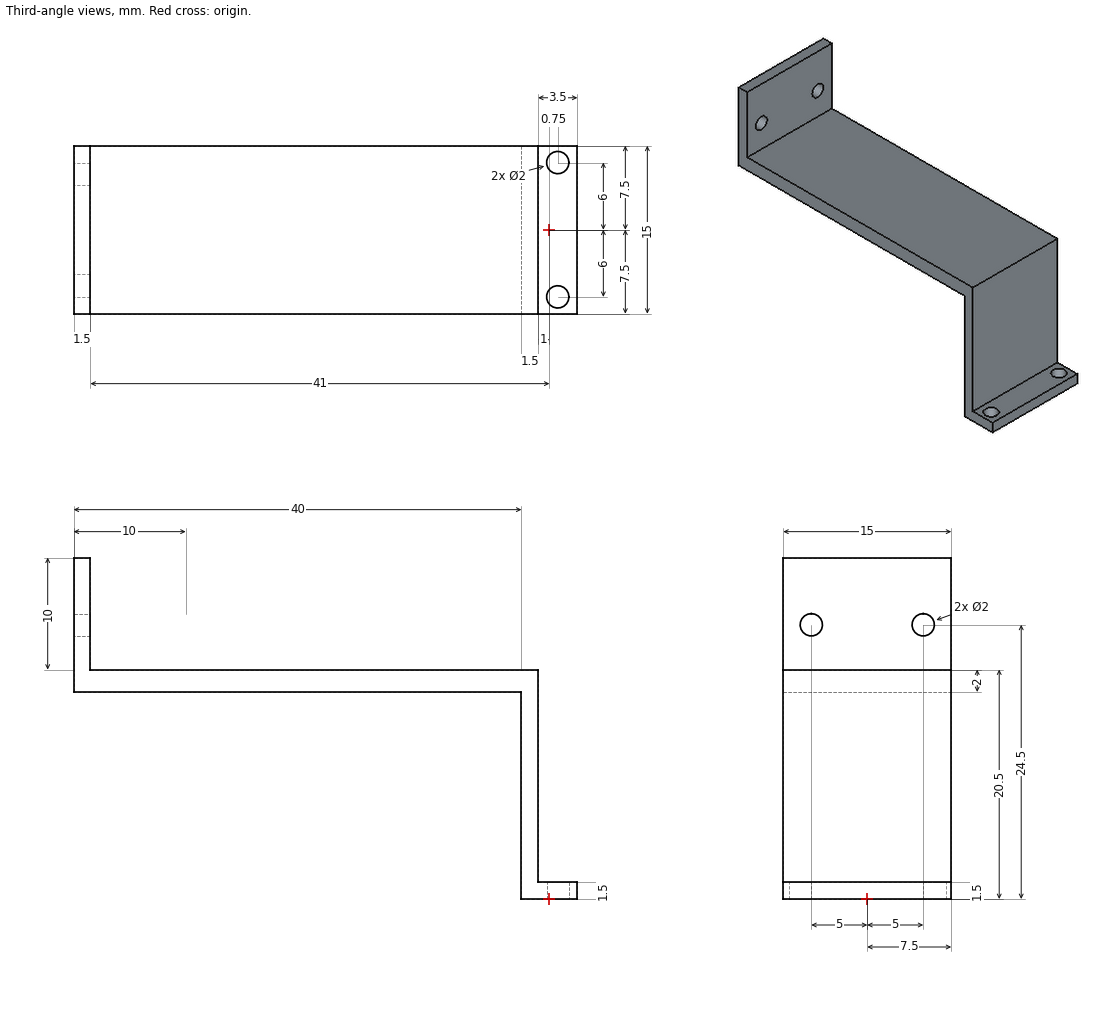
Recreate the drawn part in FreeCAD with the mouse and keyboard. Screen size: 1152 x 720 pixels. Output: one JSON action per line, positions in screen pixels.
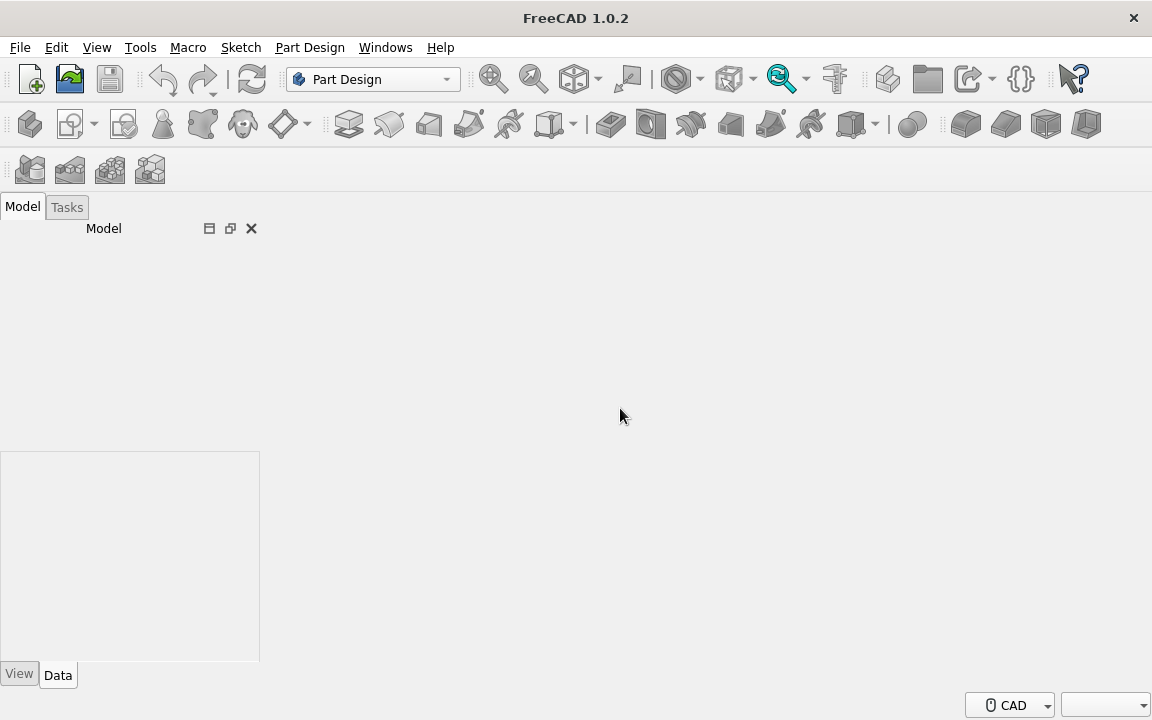
{"action": "left_click", "coordinate": [30, 80]}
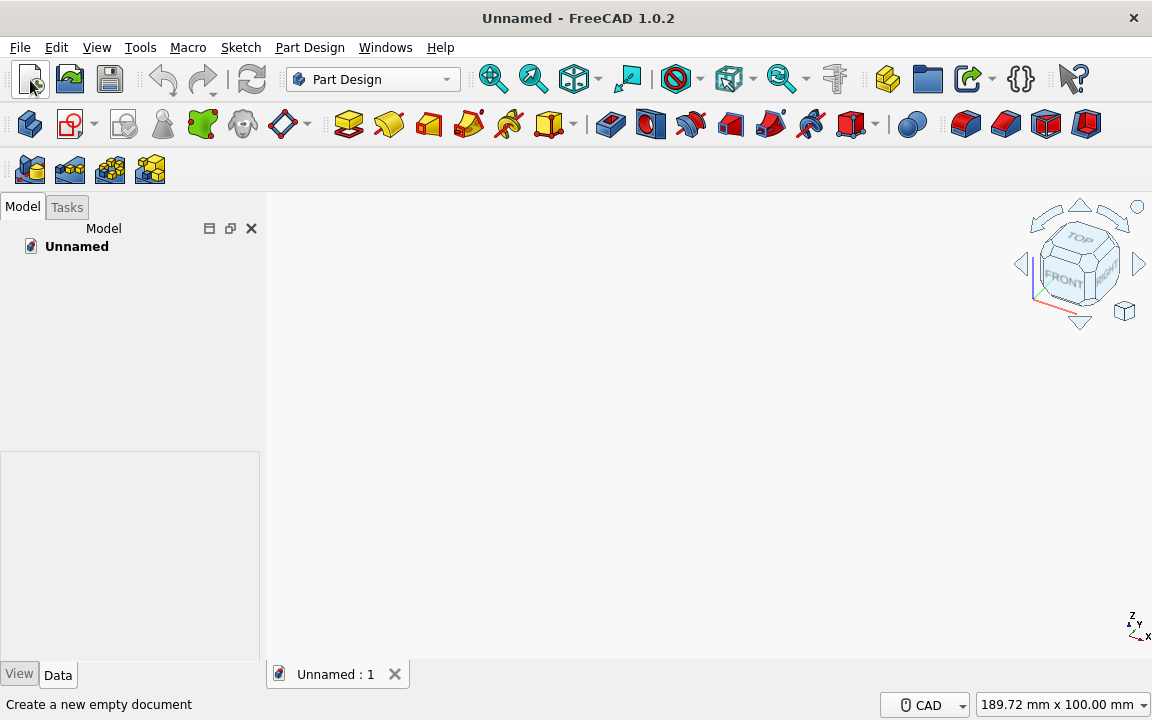
{"action": "left_click", "coordinate": [70, 124]}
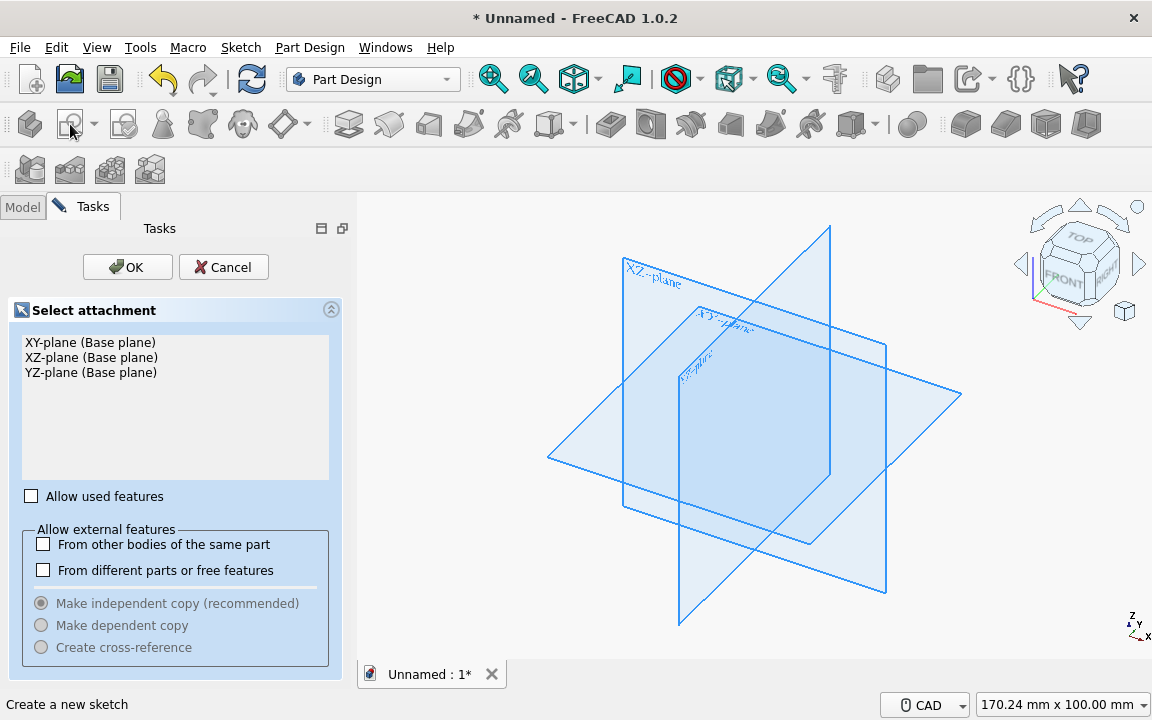
{"action": "left_click", "coordinate": [82, 342]}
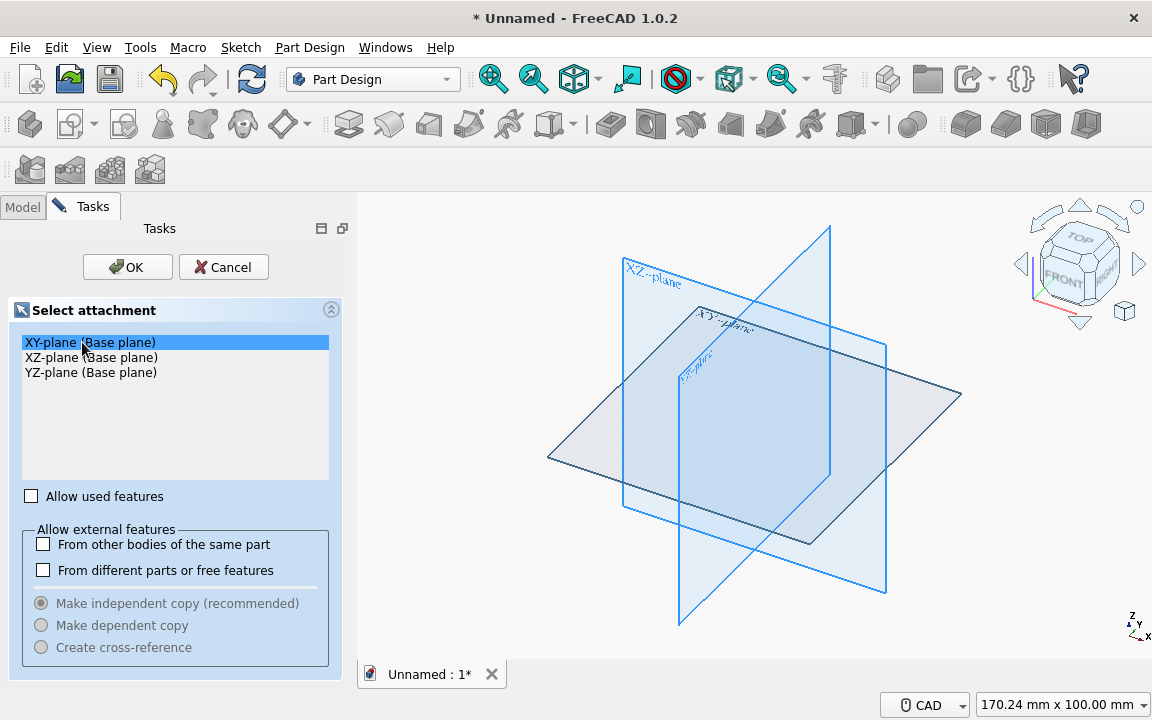
{"action": "left_click", "coordinate": [128, 267]}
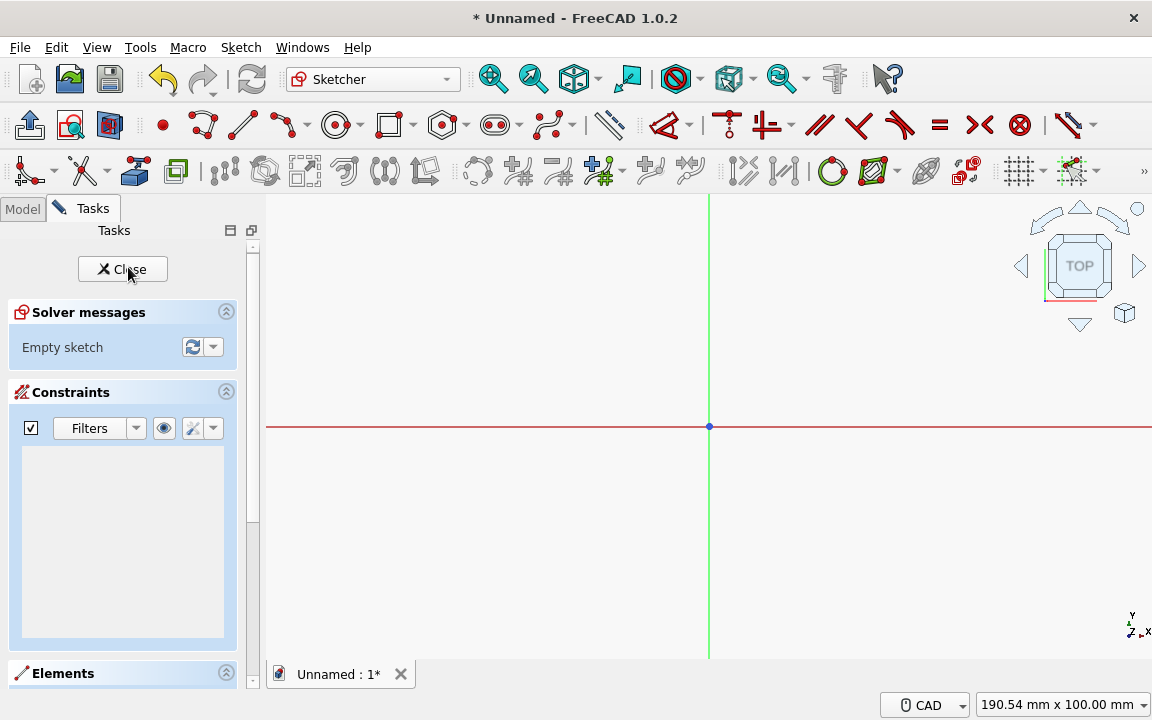
{"action": "scroll", "coordinate": [724, 426], "scroll_direction": "up", "scroll_amount": 7}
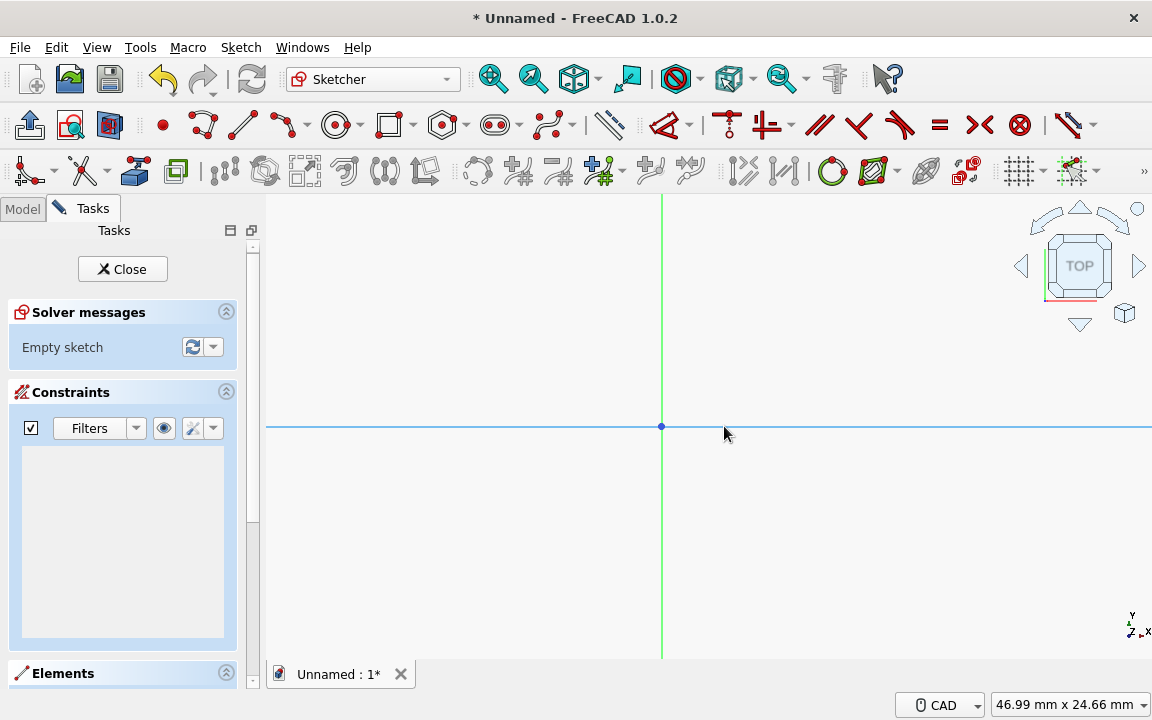
{"action": "key", "text": "g r"}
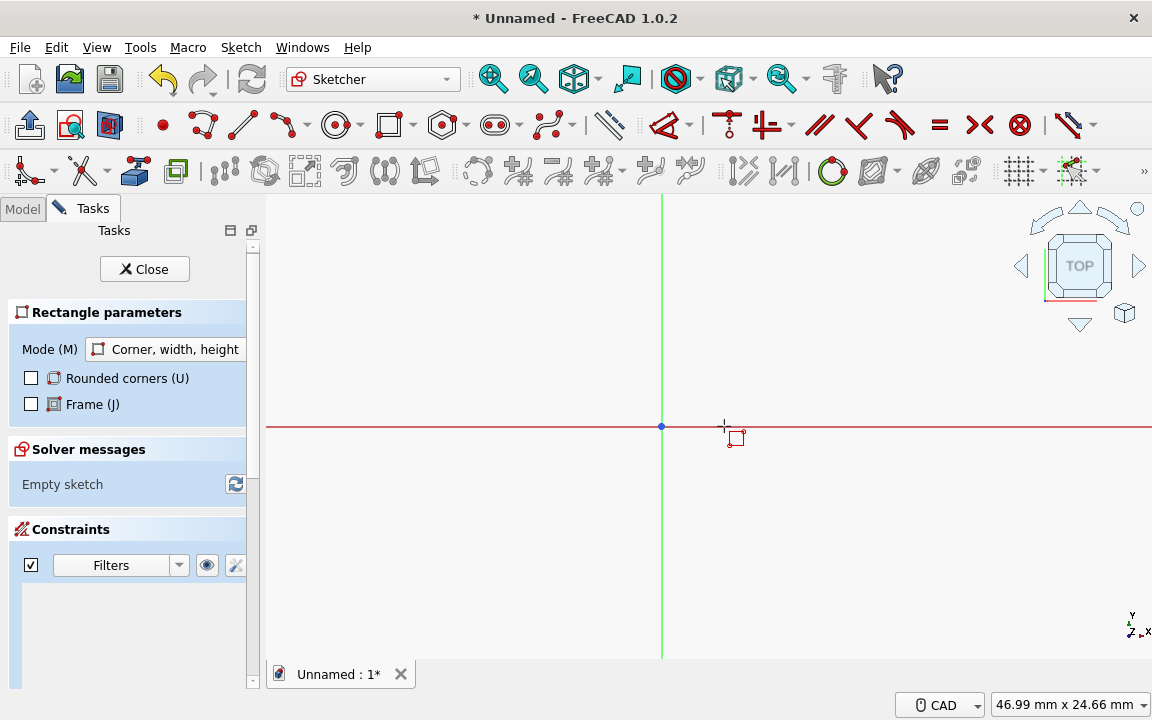
{"action": "left_click", "coordinate": [614, 285]}
{"action": "left_click", "coordinate": [643, 568]}
{"action": "key", "text": "Escape"}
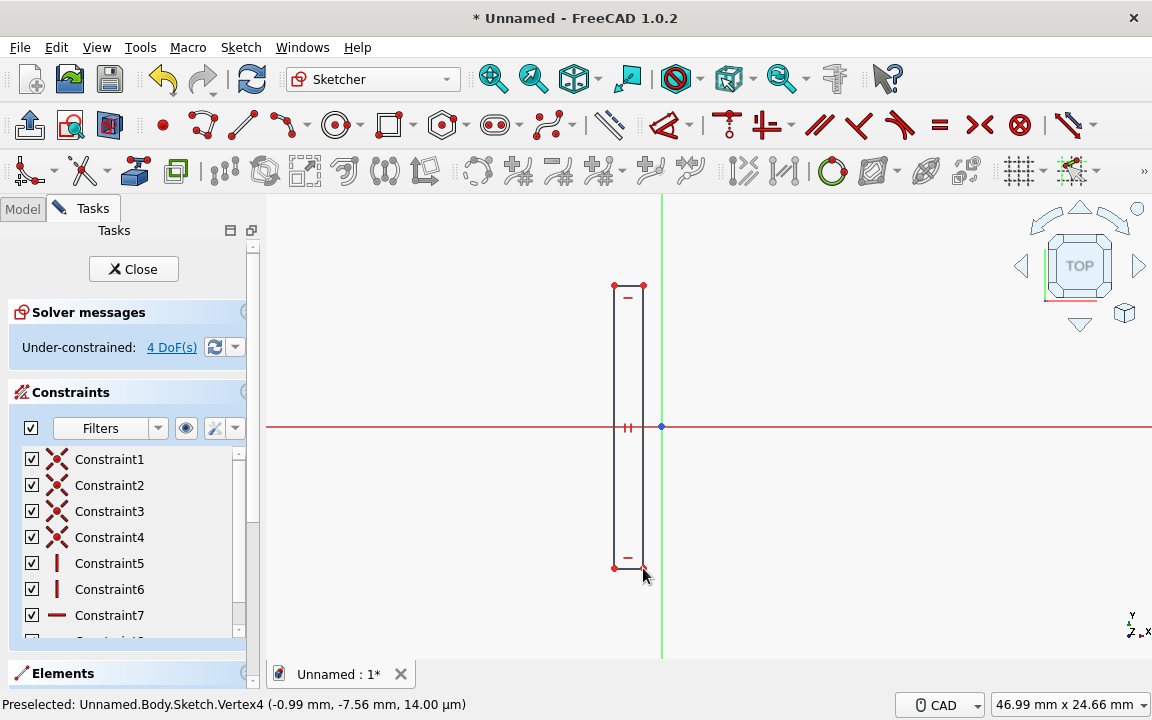
{"action": "left_click", "coordinate": [664, 126]}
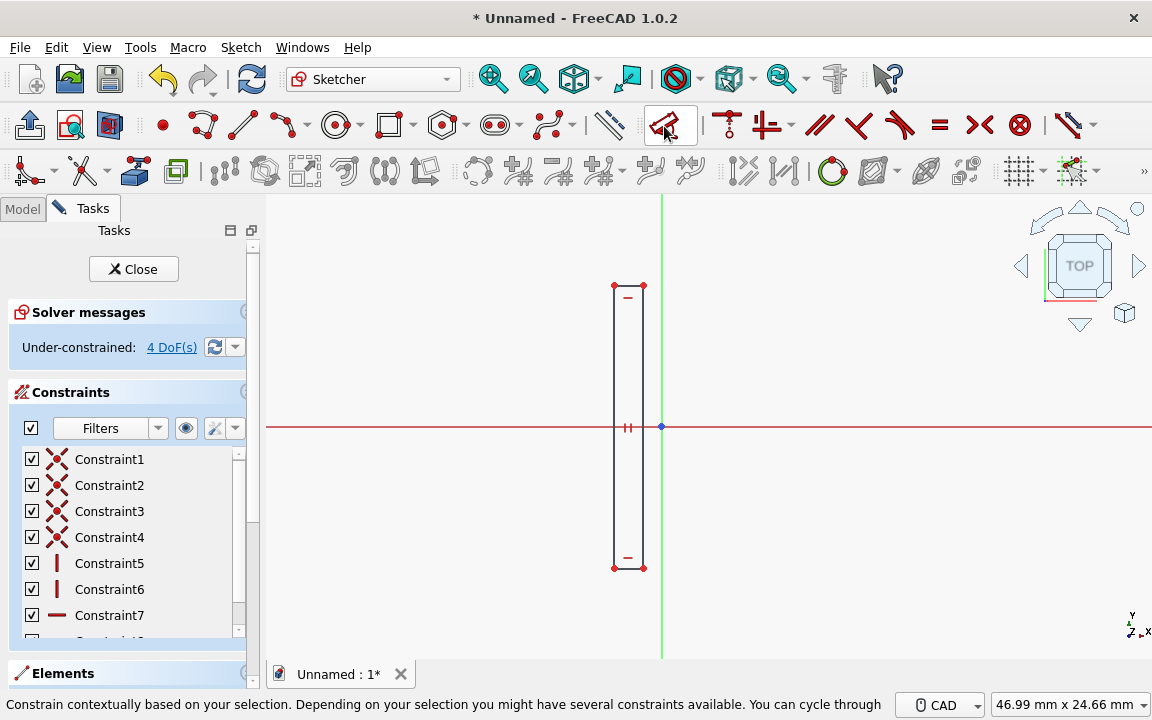
{"action": "left_click", "coordinate": [614, 371]}
{"action": "left_click", "coordinate": [580, 362]}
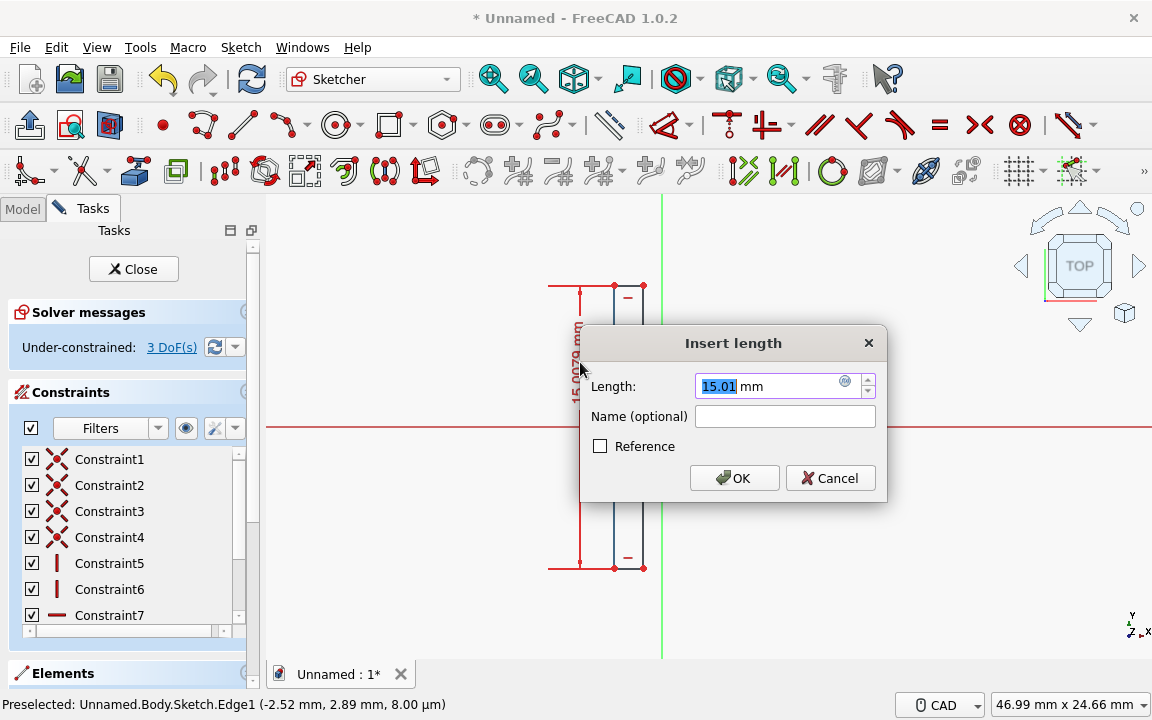
{"action": "type", "text": "15"}
{"action": "key", "text": "Return"}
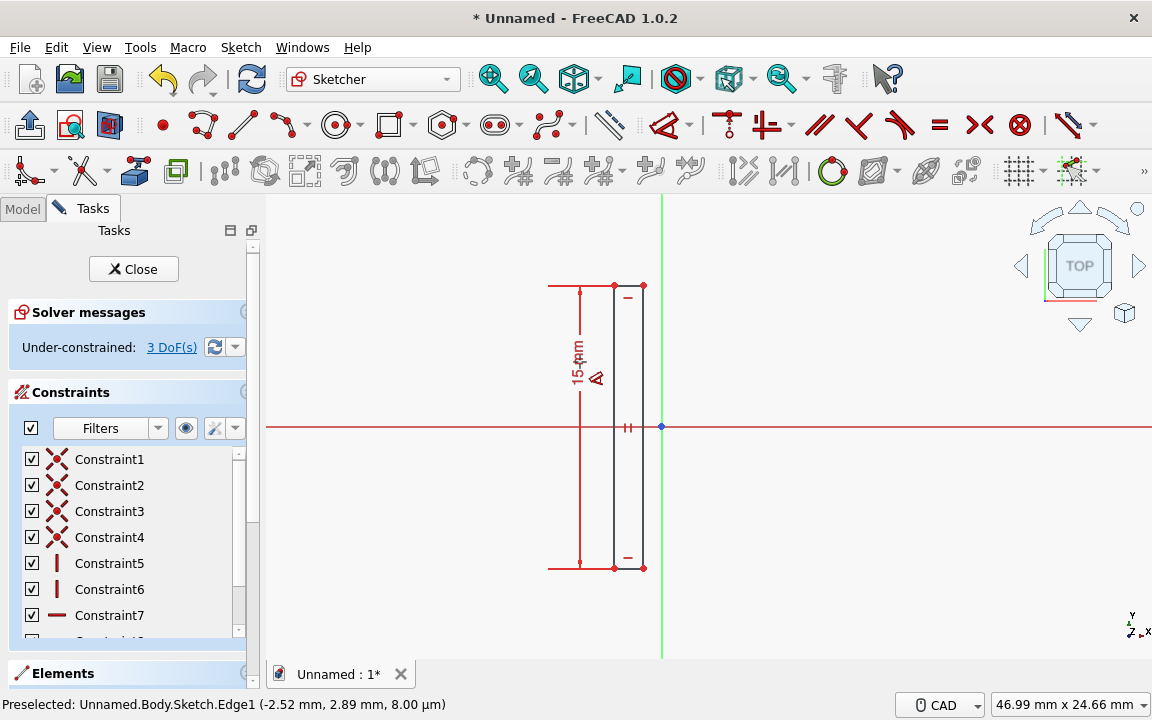
{"action": "scroll", "coordinate": [643, 569], "scroll_direction": "up", "scroll_amount": 4}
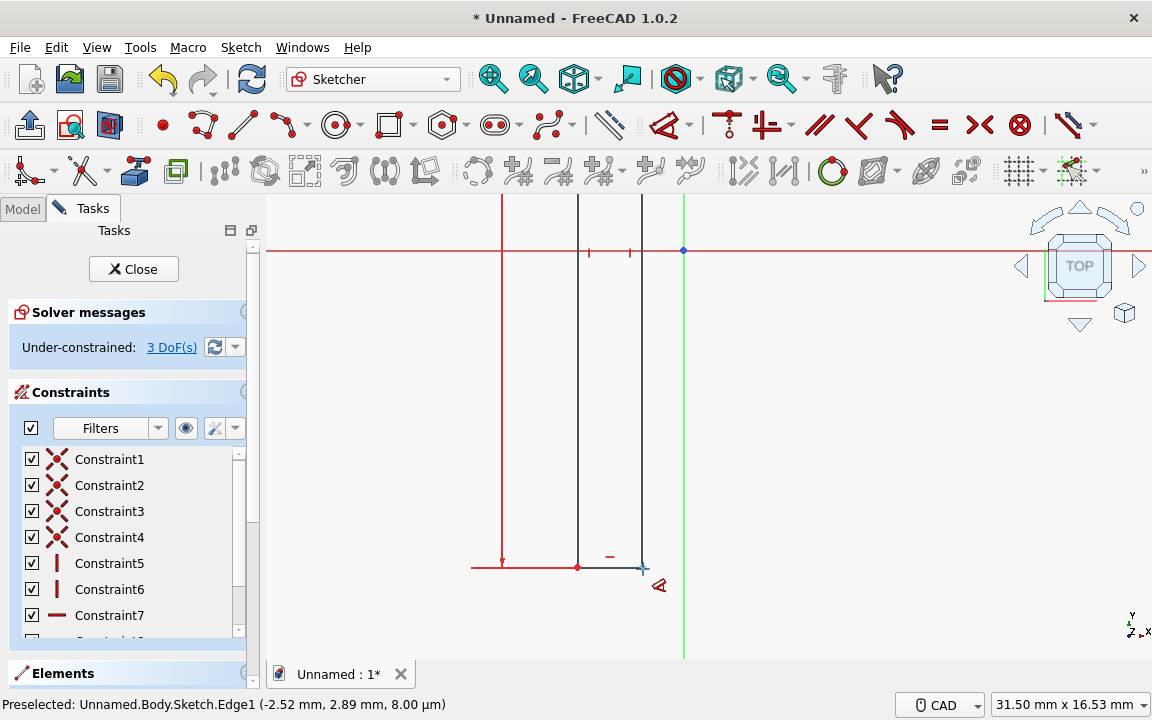
{"action": "left_click", "coordinate": [642, 568]}
{"action": "left_click", "coordinate": [663, 602]}